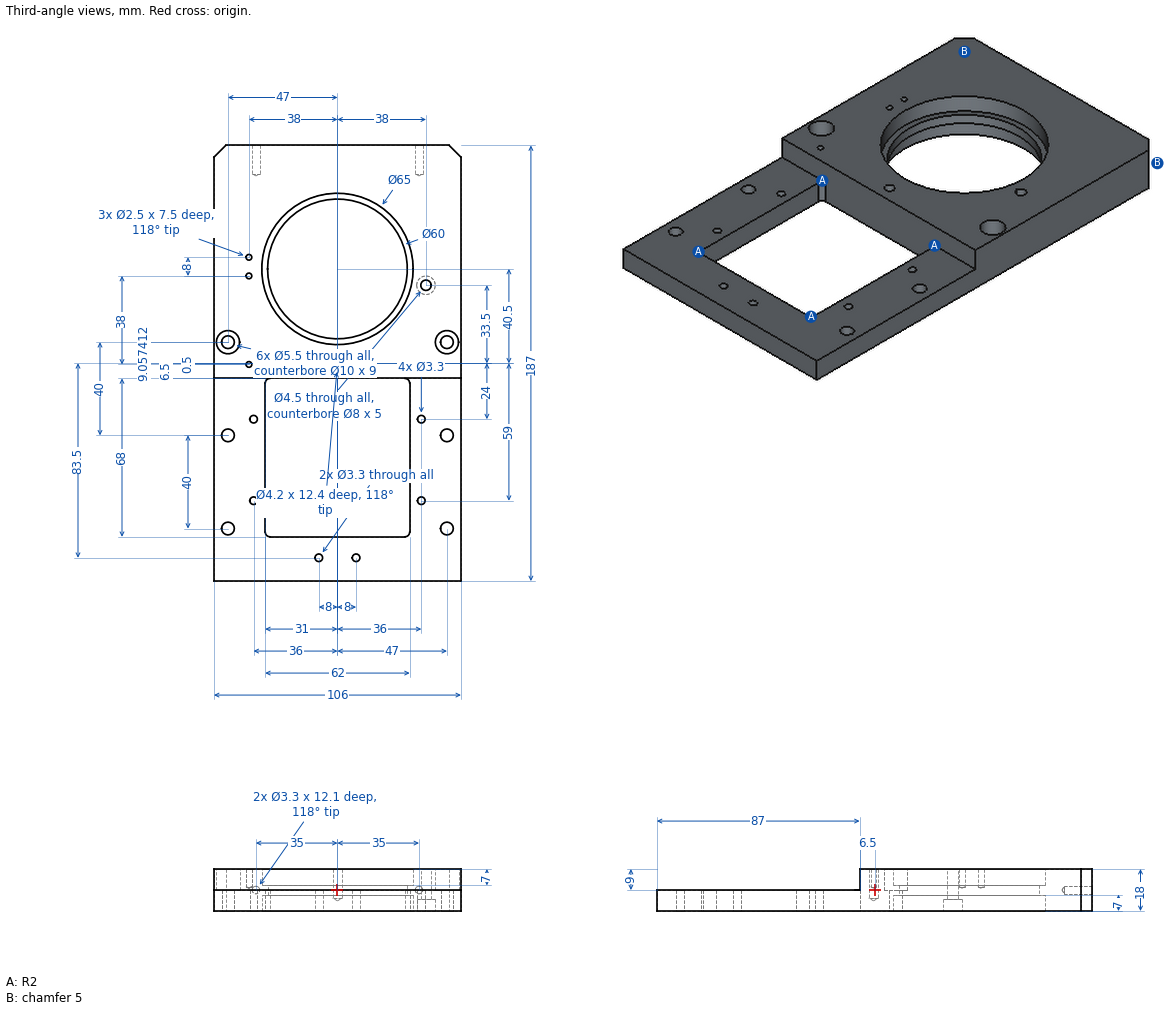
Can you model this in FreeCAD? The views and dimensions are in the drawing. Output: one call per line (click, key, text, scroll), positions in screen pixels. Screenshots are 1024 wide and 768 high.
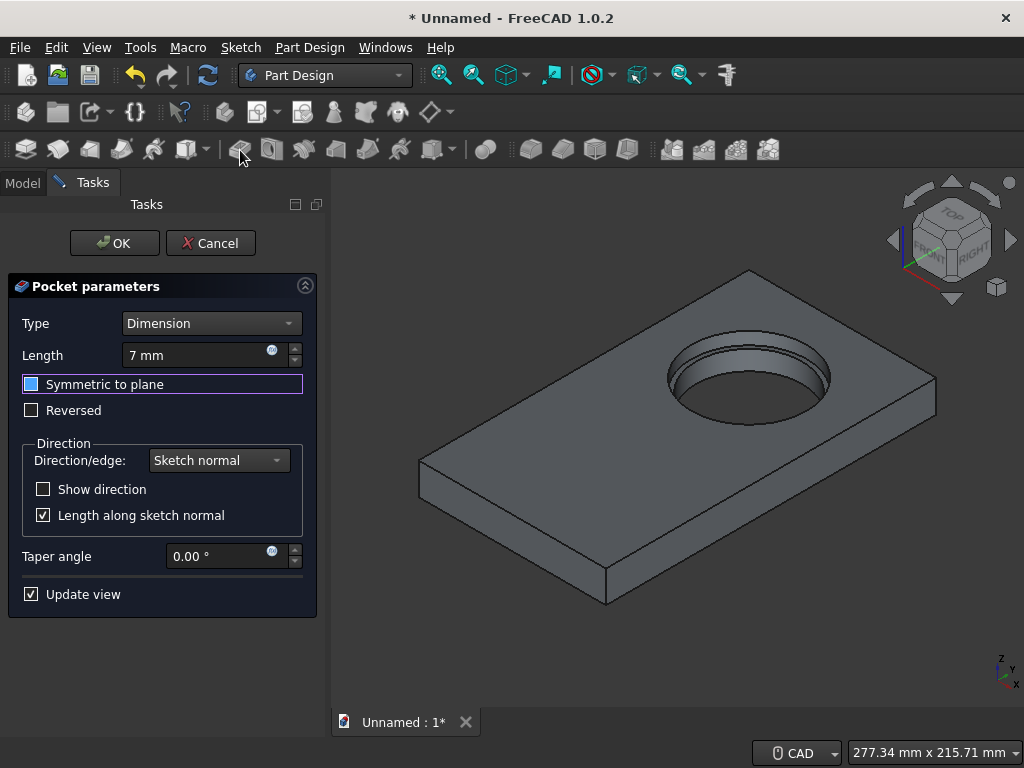
click(115, 243)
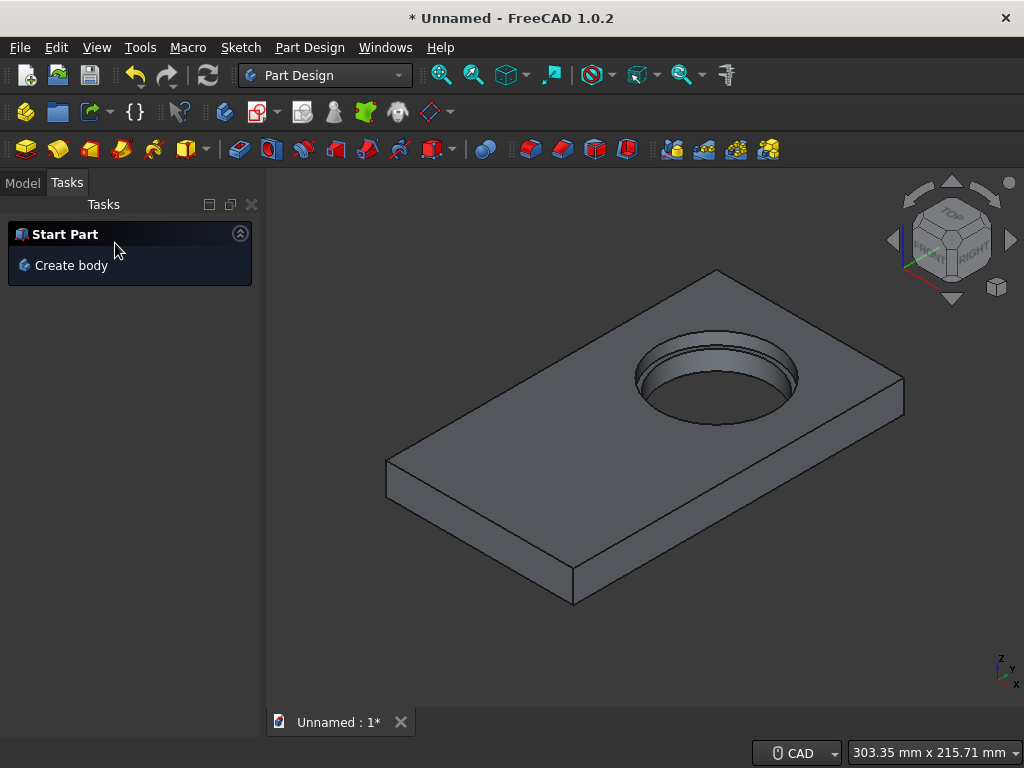
click(23, 182)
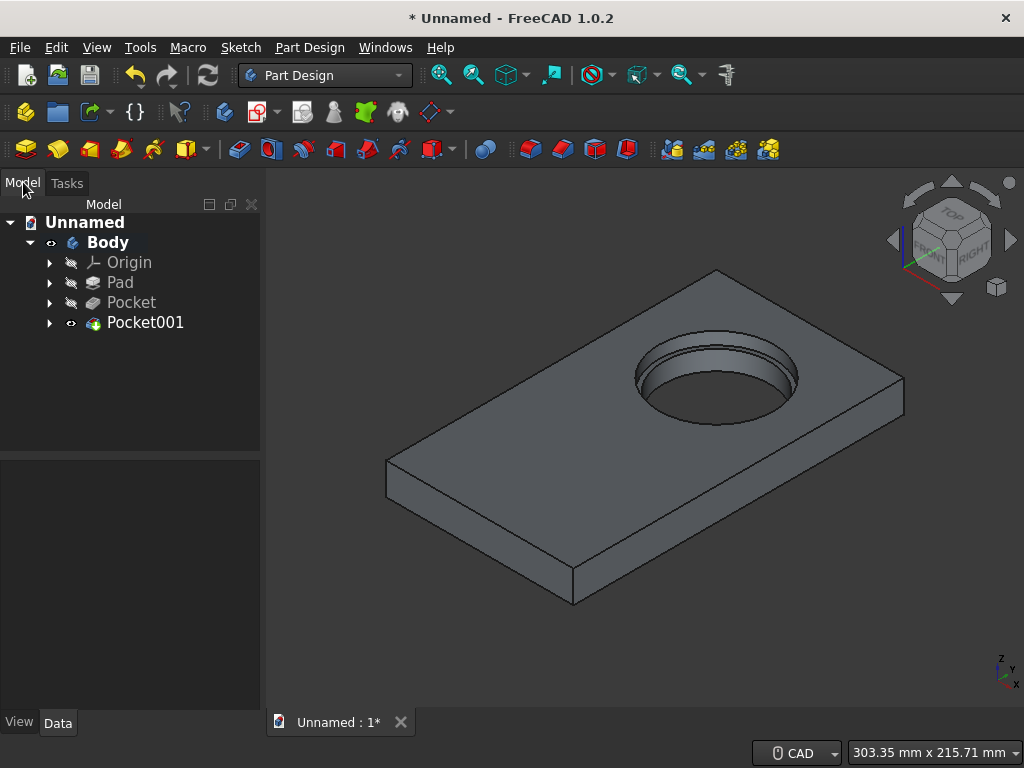
click(50, 263)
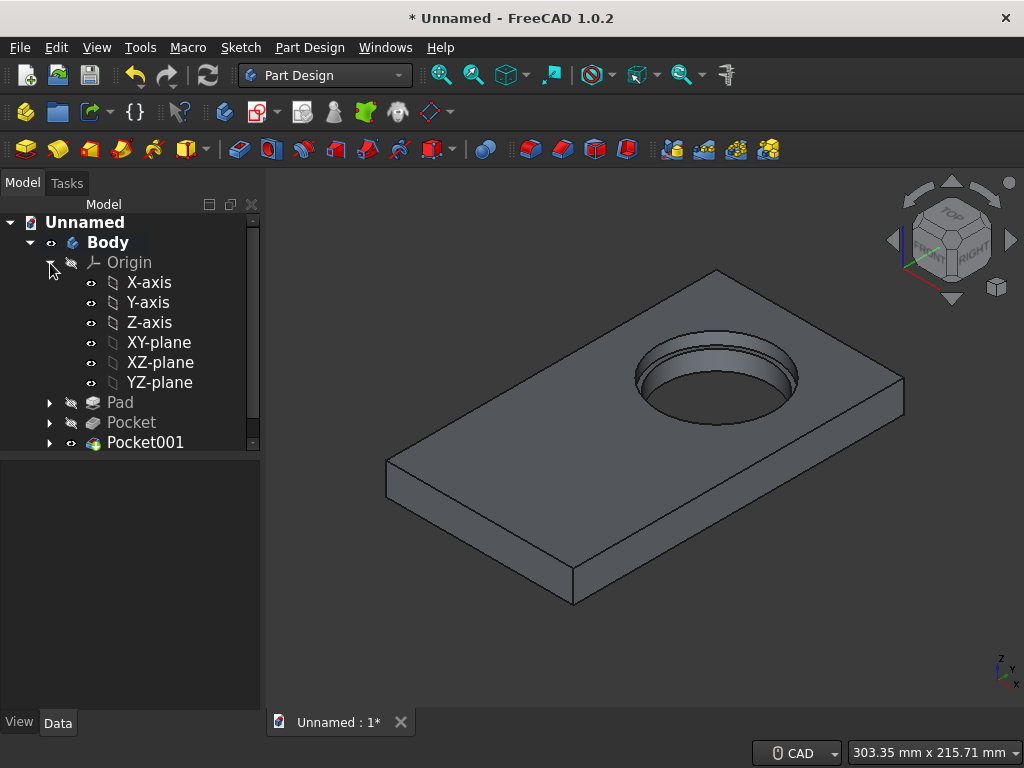
click(136, 343)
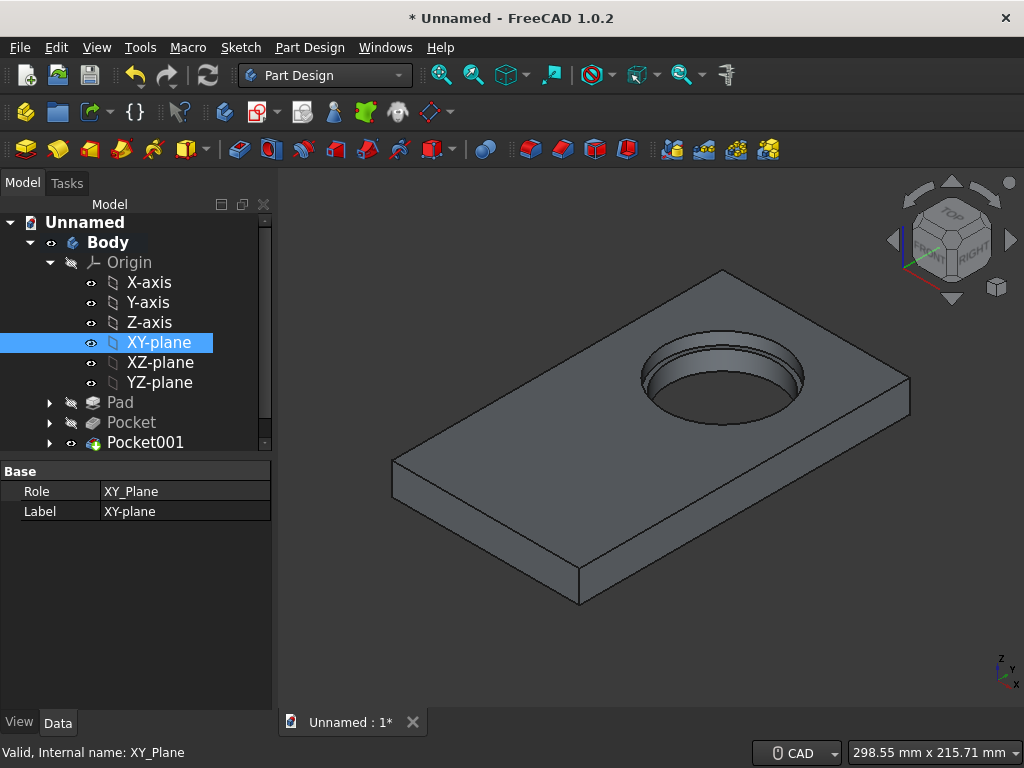
click(430, 112)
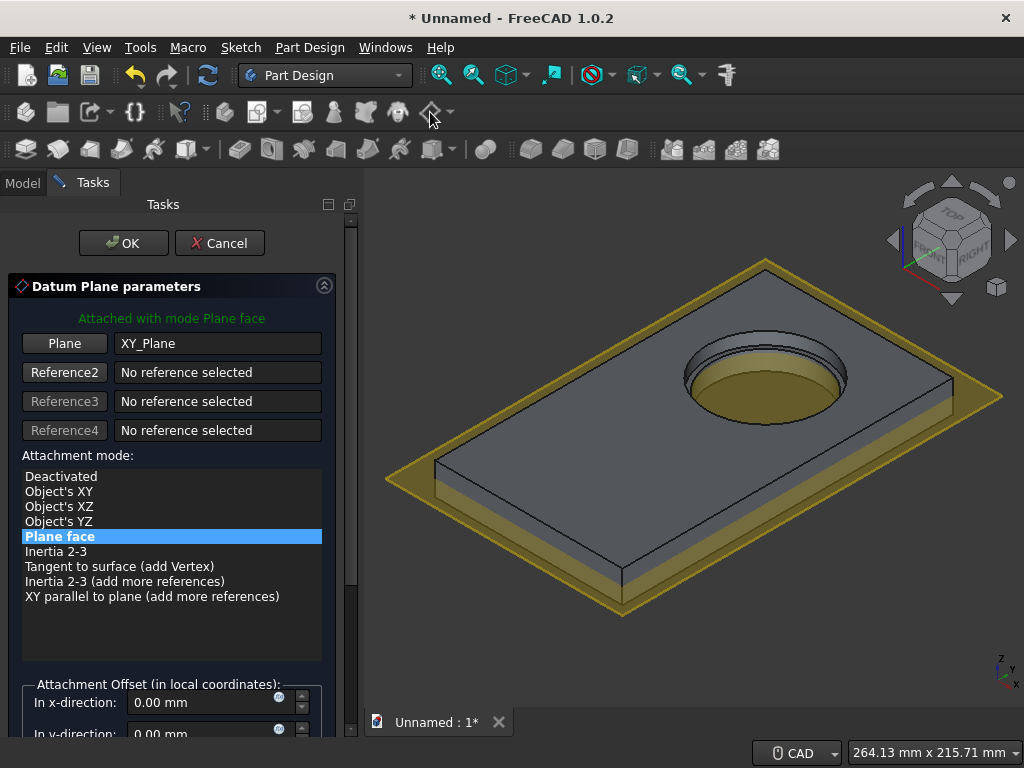
scroll(351, 475, down, 2)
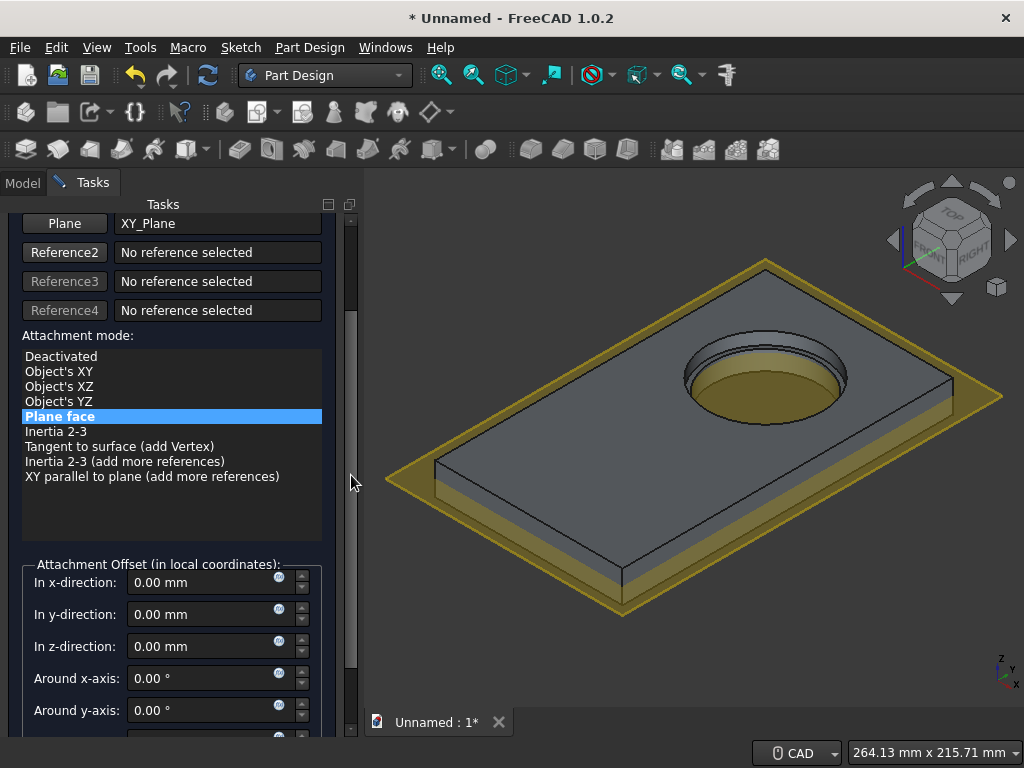
triple_click(210, 646)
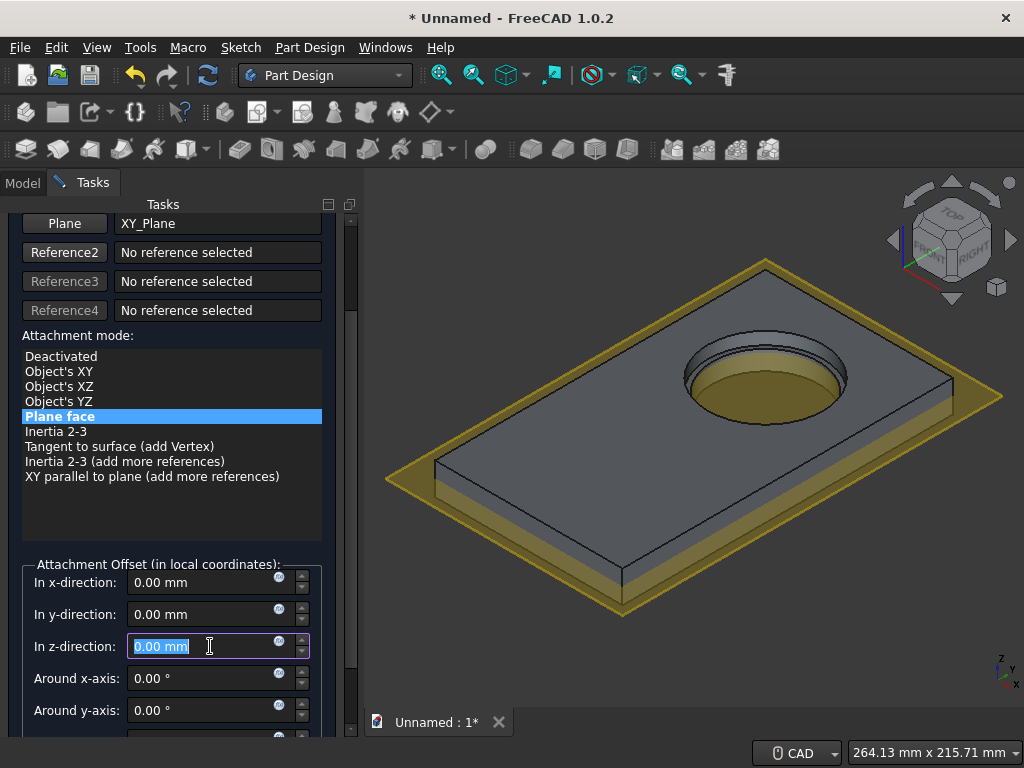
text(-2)
key(Tab)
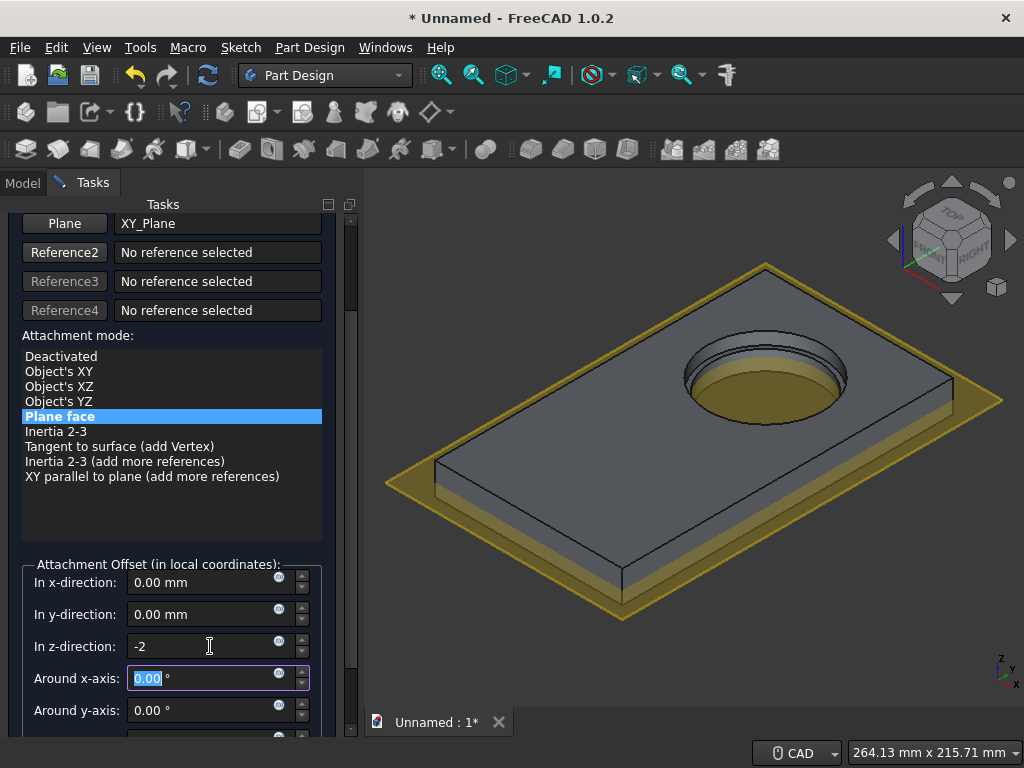
scroll(351, 475, up, 3)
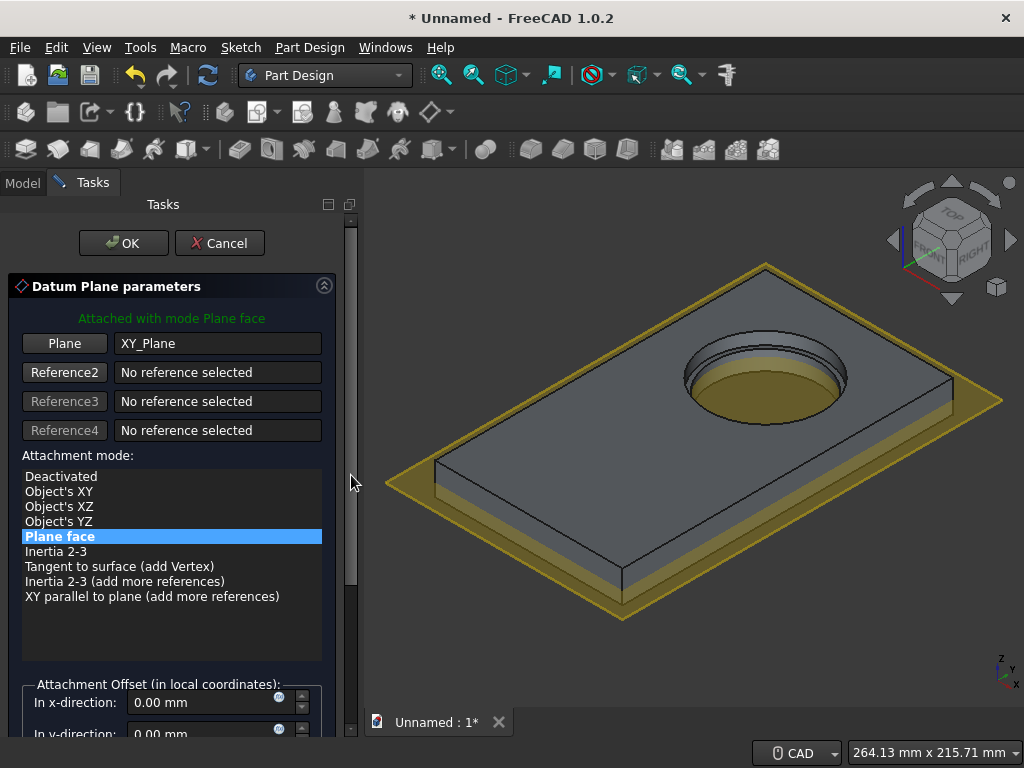
click(124, 243)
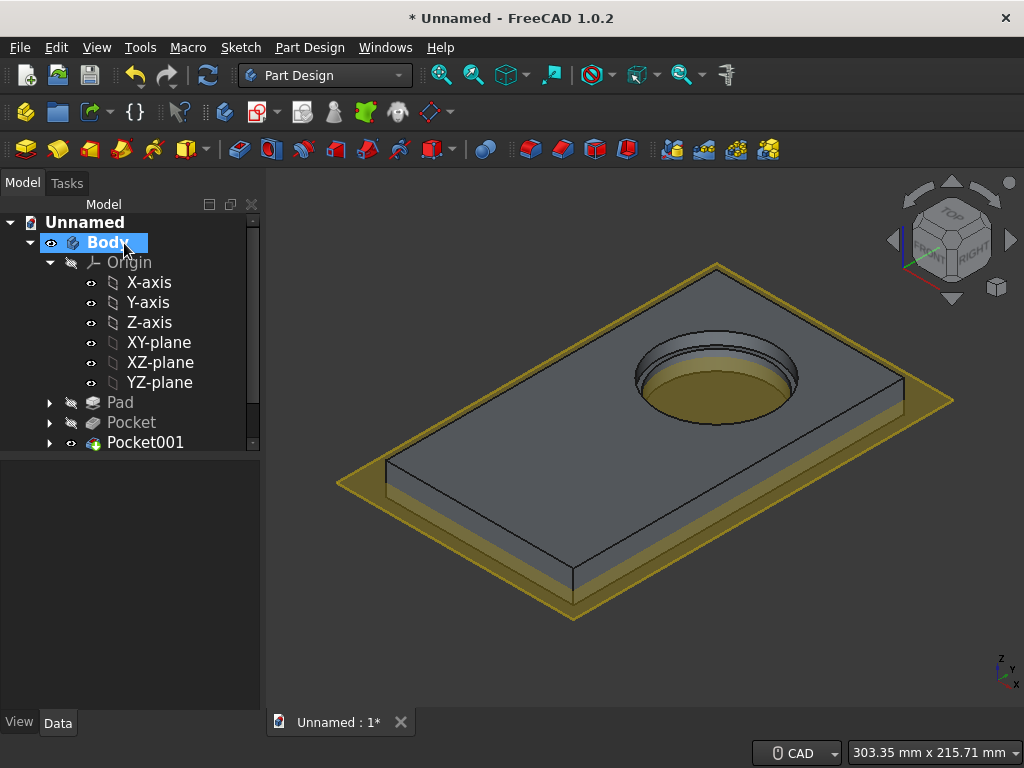
scroll(100, 338, down, 3)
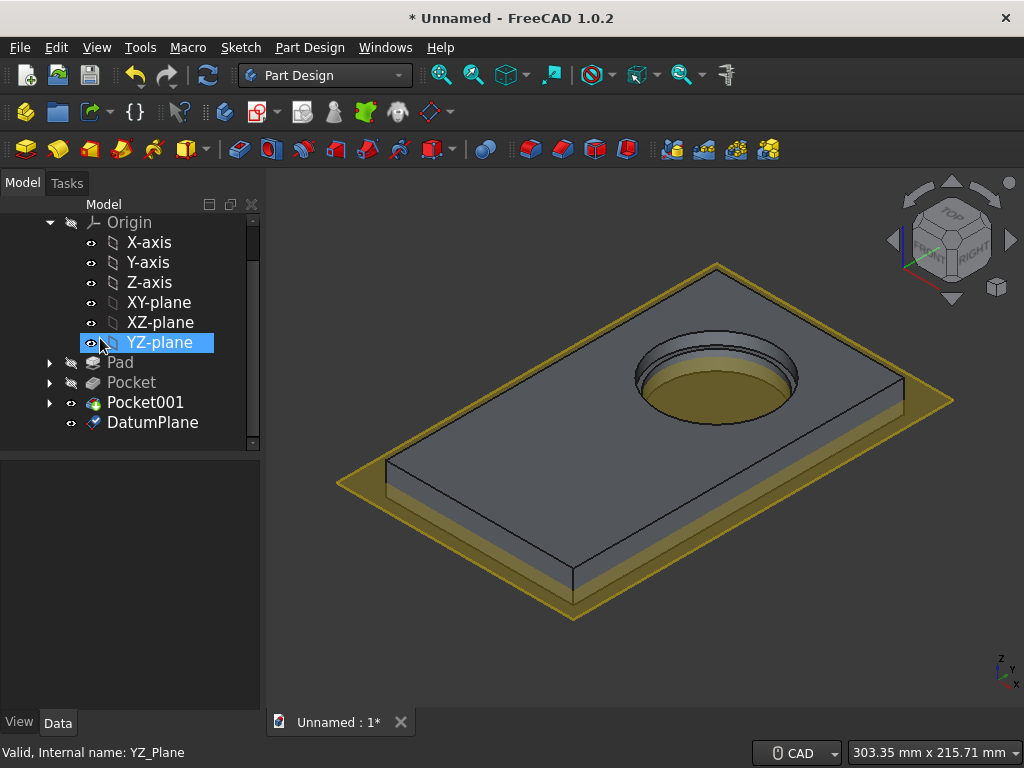
click(116, 423)